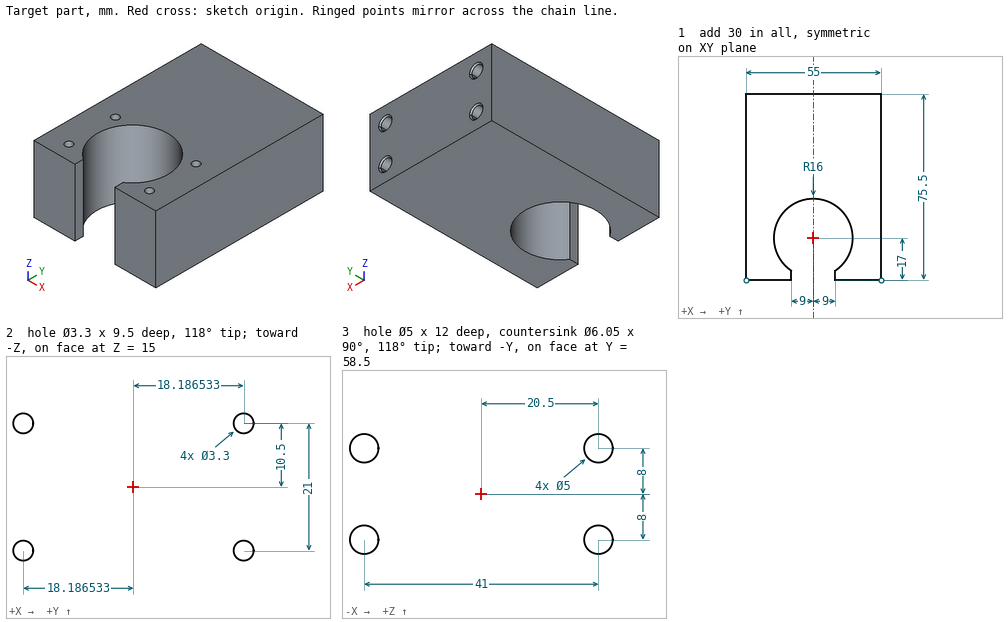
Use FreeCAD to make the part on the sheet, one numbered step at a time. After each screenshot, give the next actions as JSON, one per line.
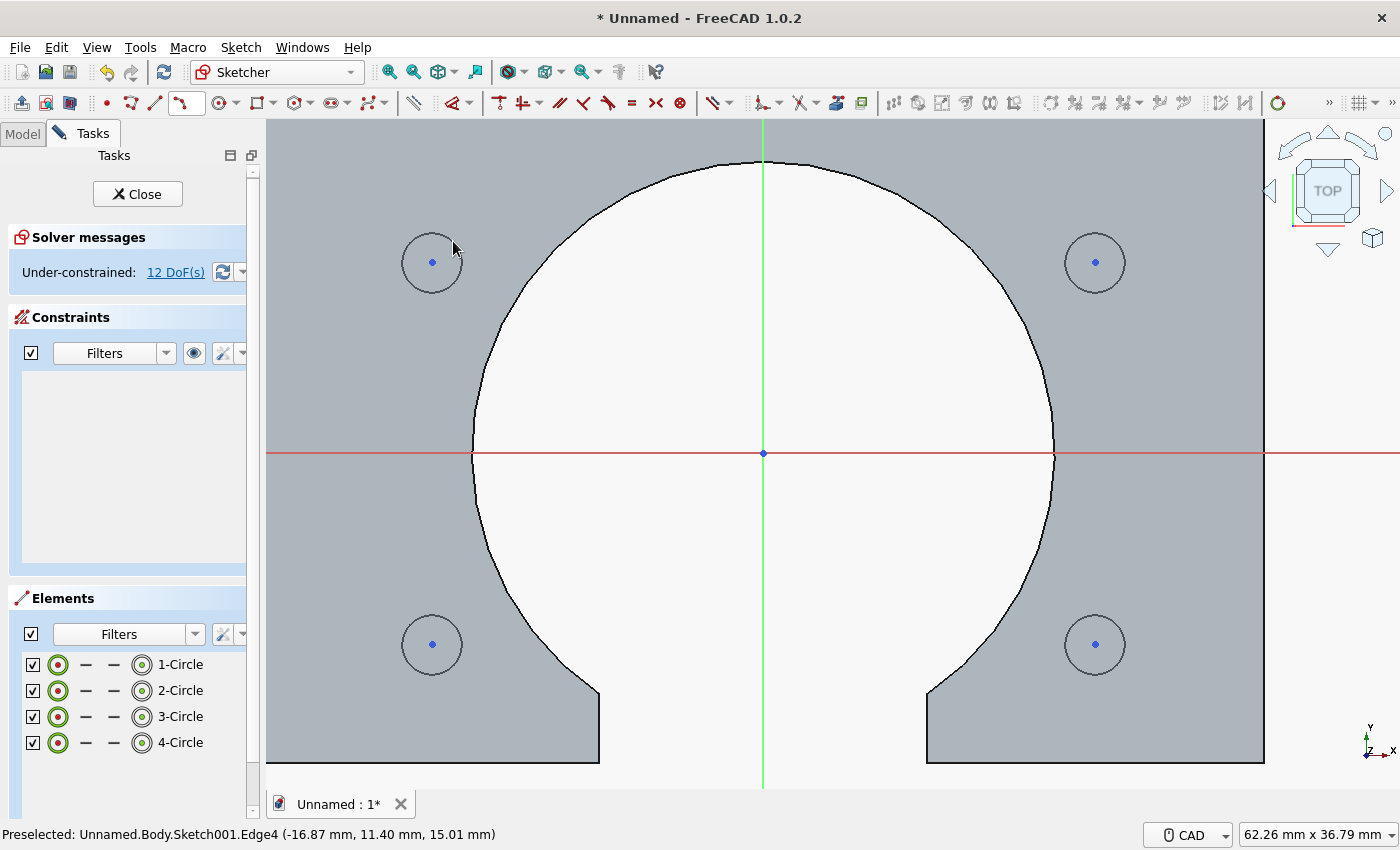
{"action": "left_click", "coordinate": [1116, 242]}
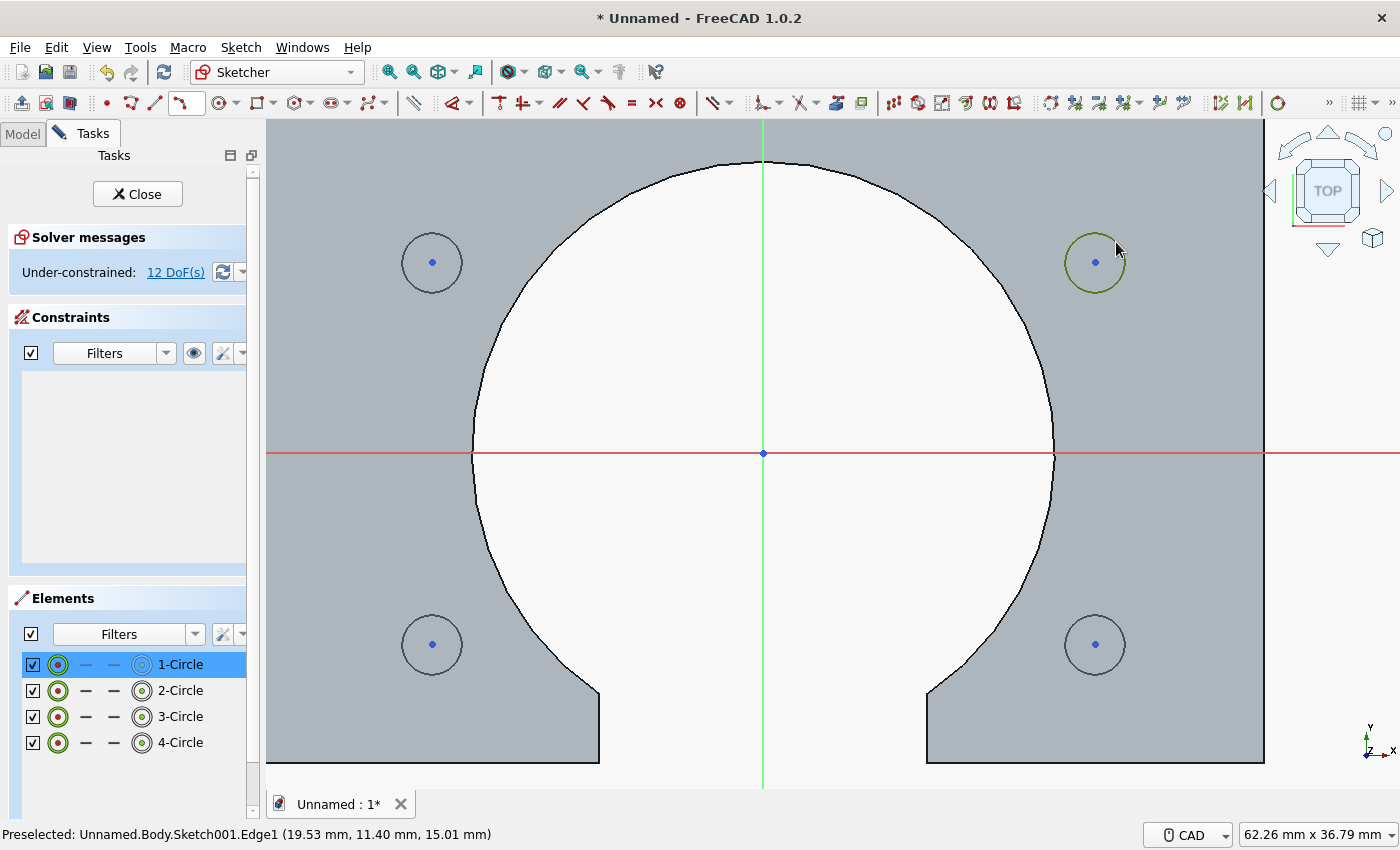
{"action": "left_click", "coordinate": [1116, 624]}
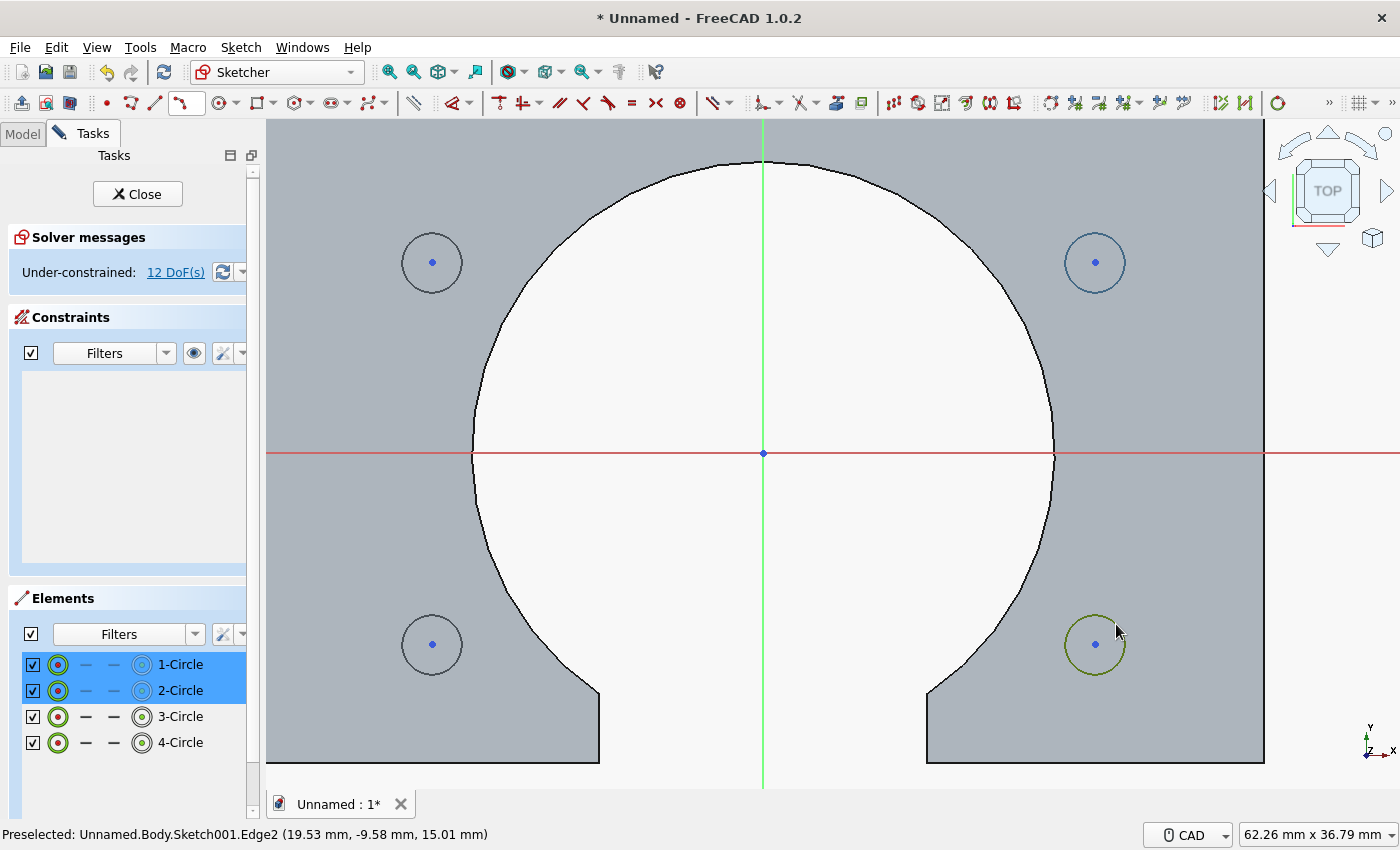
{"action": "left_click", "coordinate": [453, 624]}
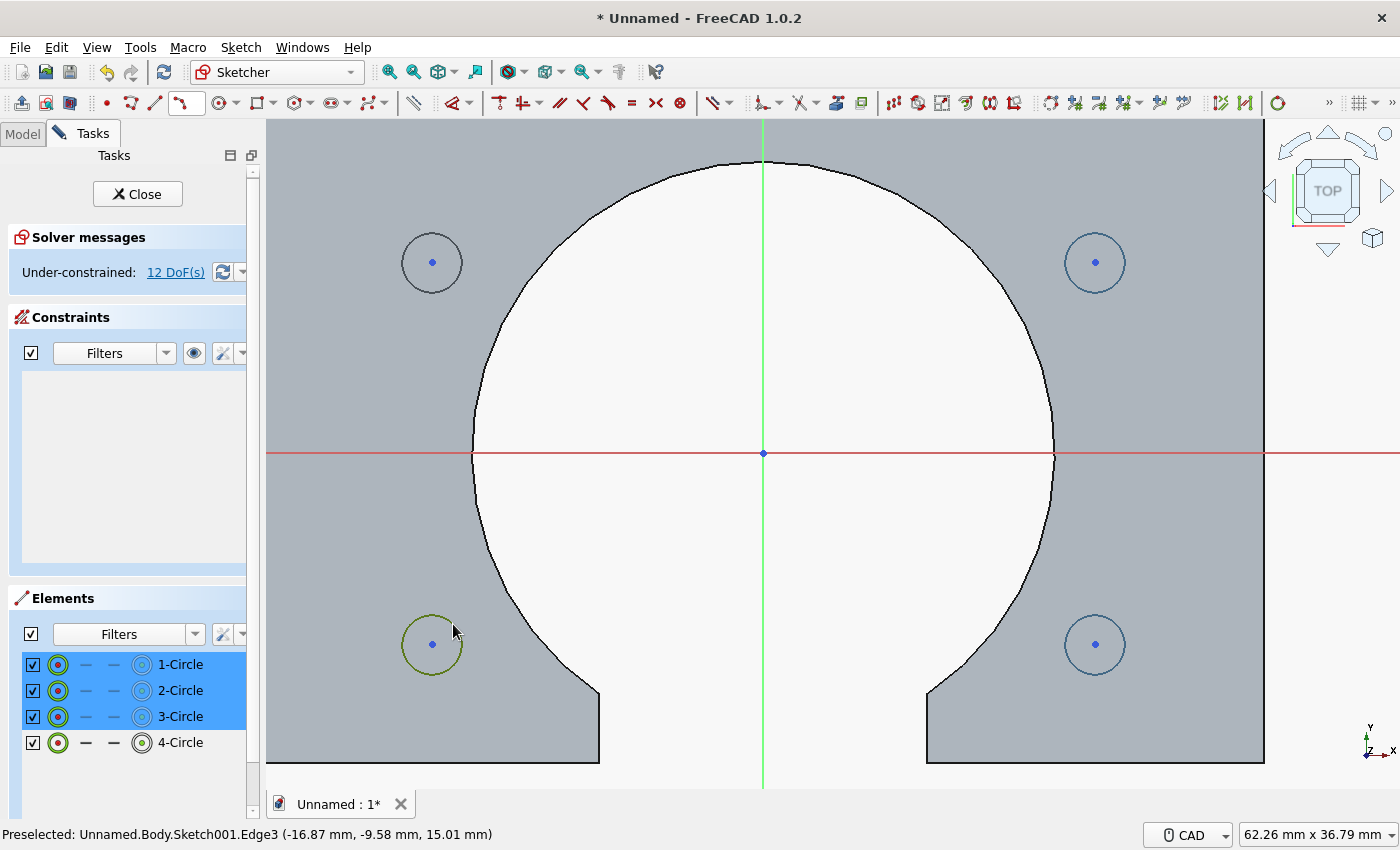
{"action": "left_click", "coordinate": [453, 242]}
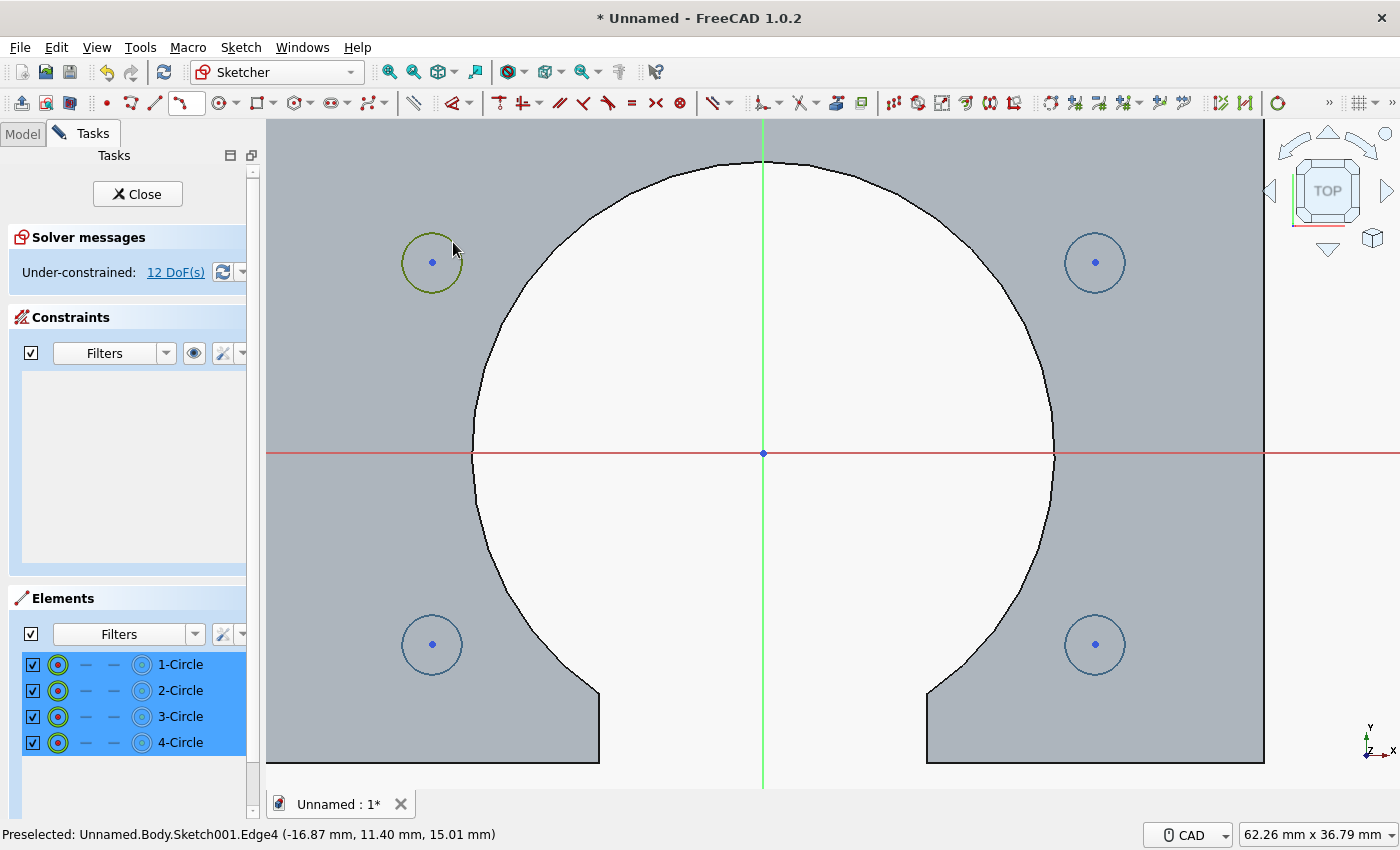
{"action": "left_click", "coordinate": [632, 104]}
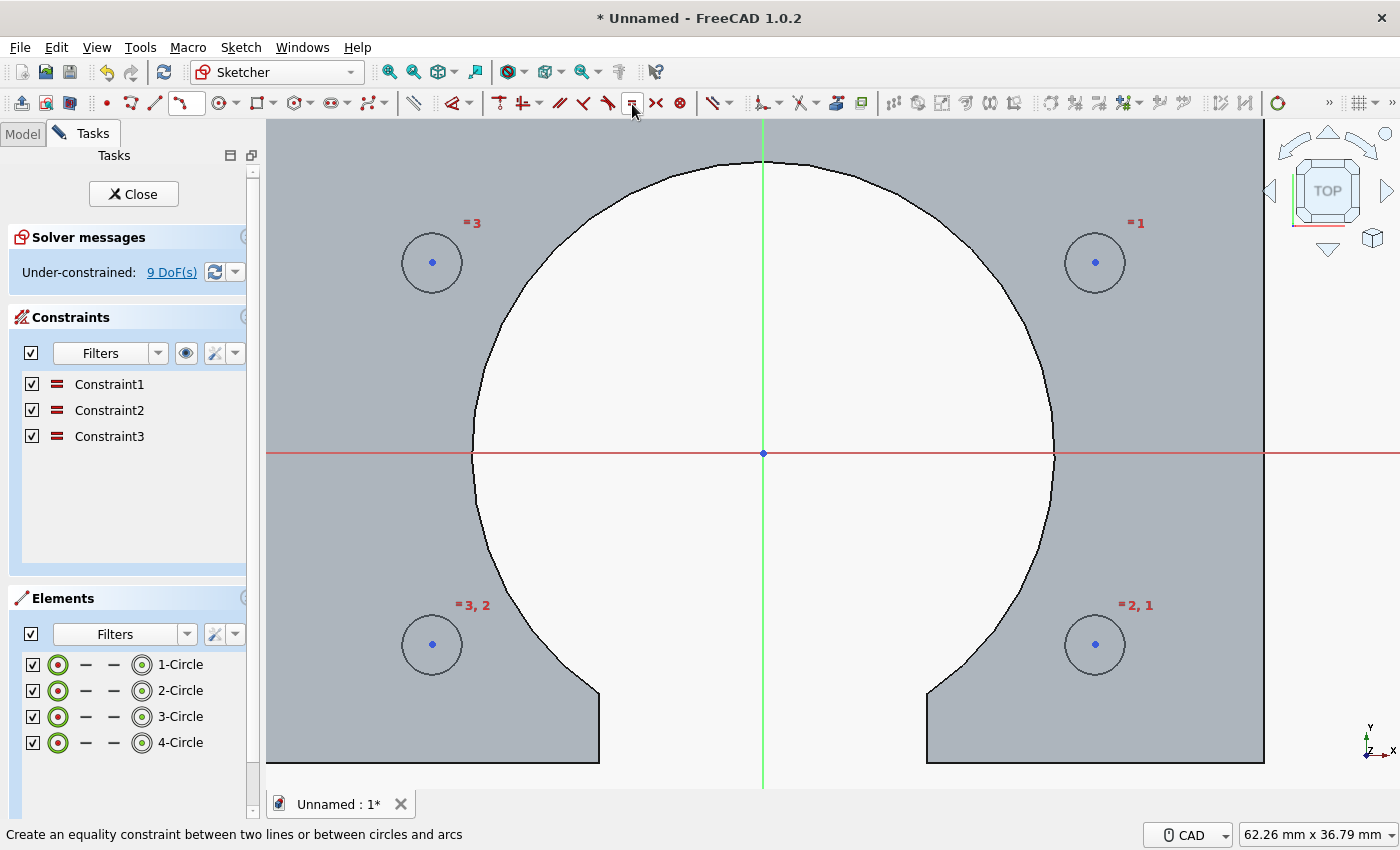
{"action": "left_click", "coordinate": [1095, 263]}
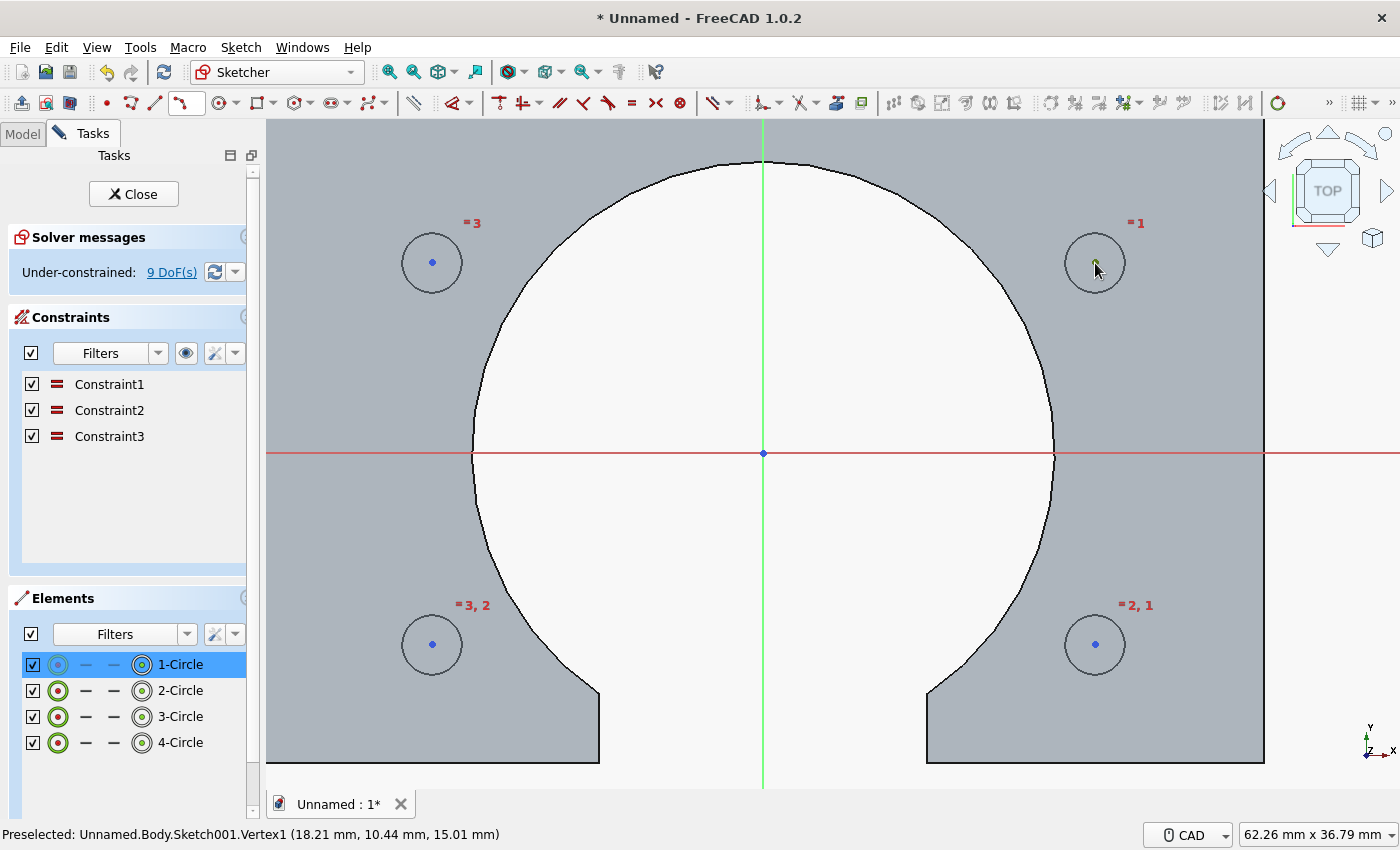
{"action": "left_click", "coordinate": [1095, 645]}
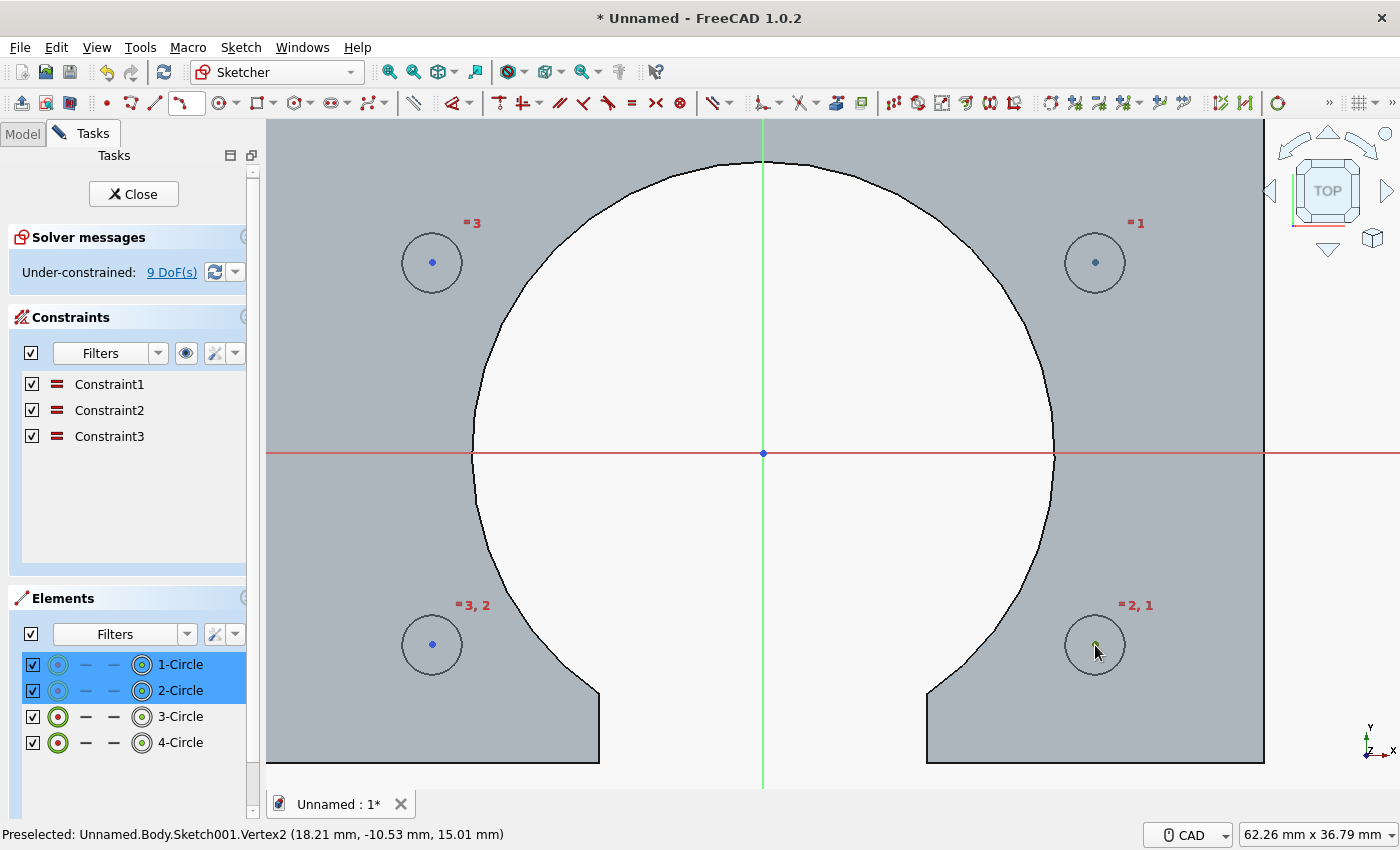
{"action": "key", "text": "v"}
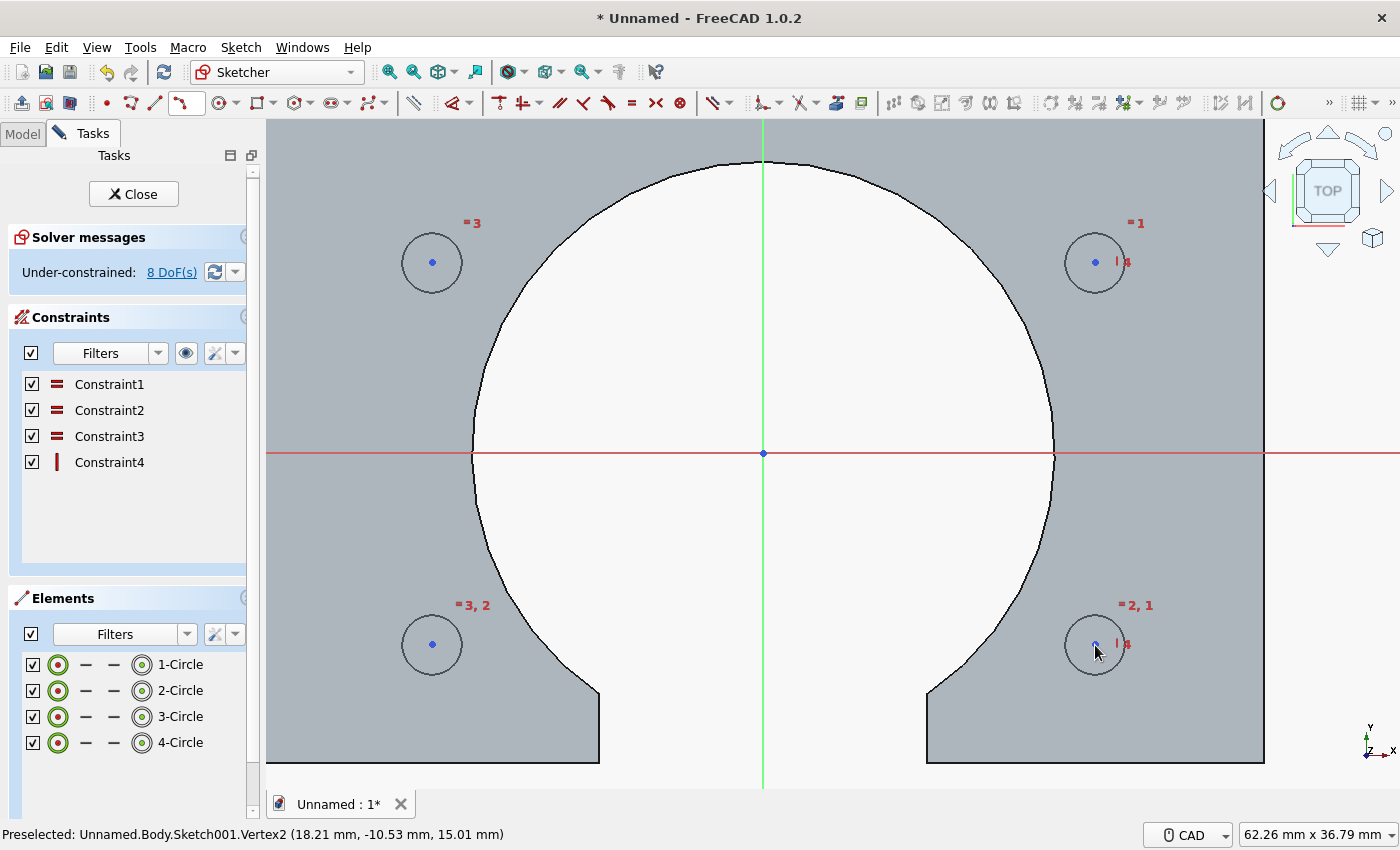
{"action": "left_click", "coordinate": [1095, 645]}